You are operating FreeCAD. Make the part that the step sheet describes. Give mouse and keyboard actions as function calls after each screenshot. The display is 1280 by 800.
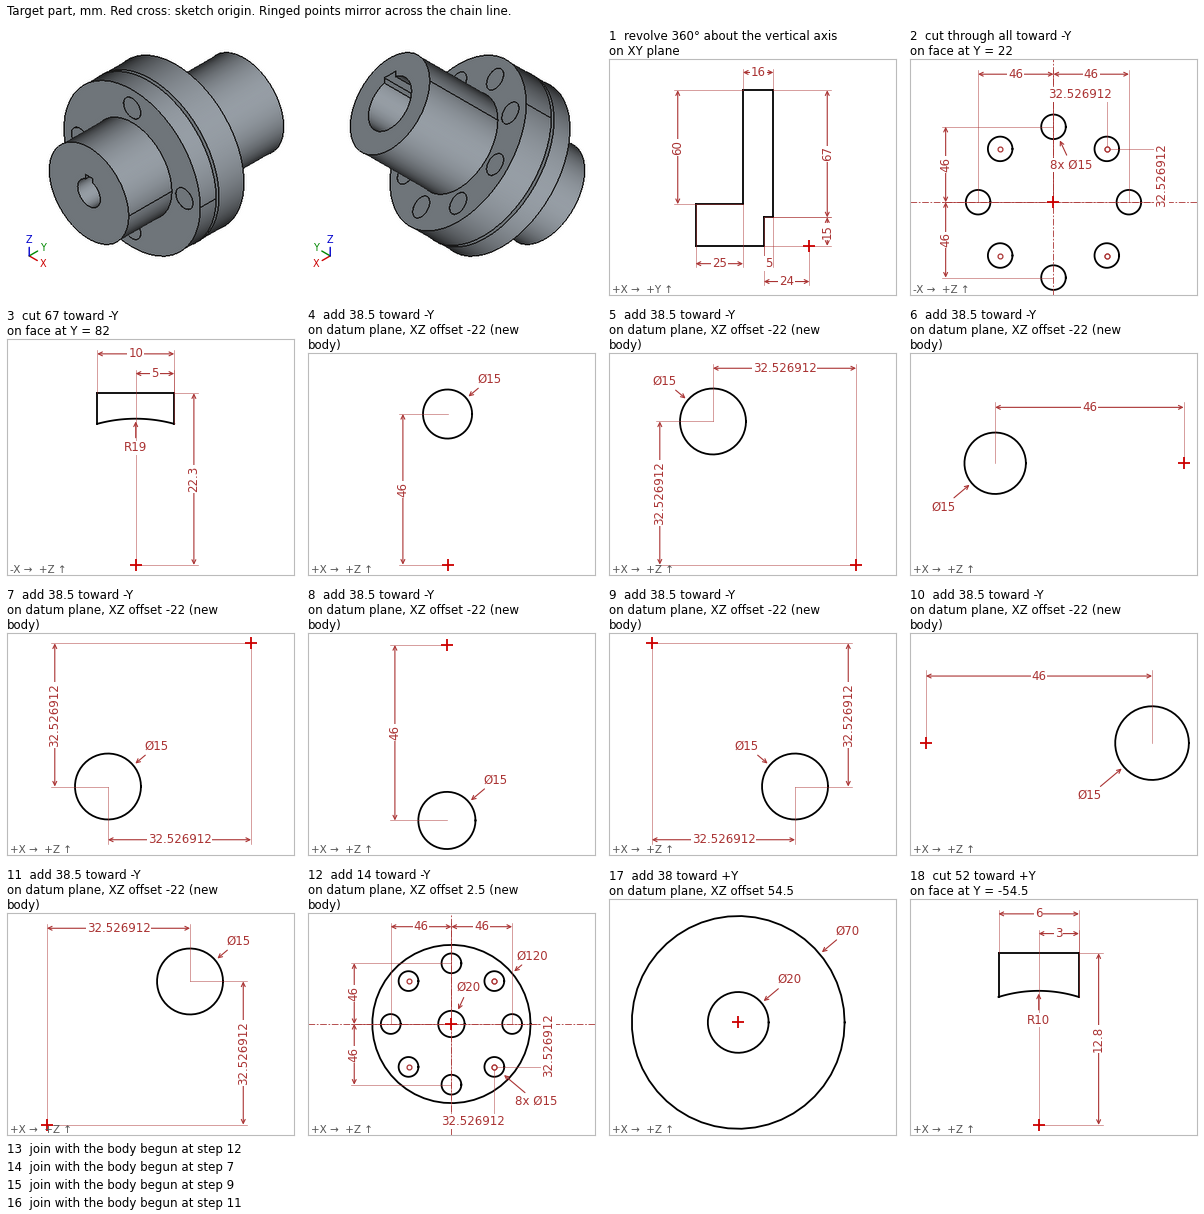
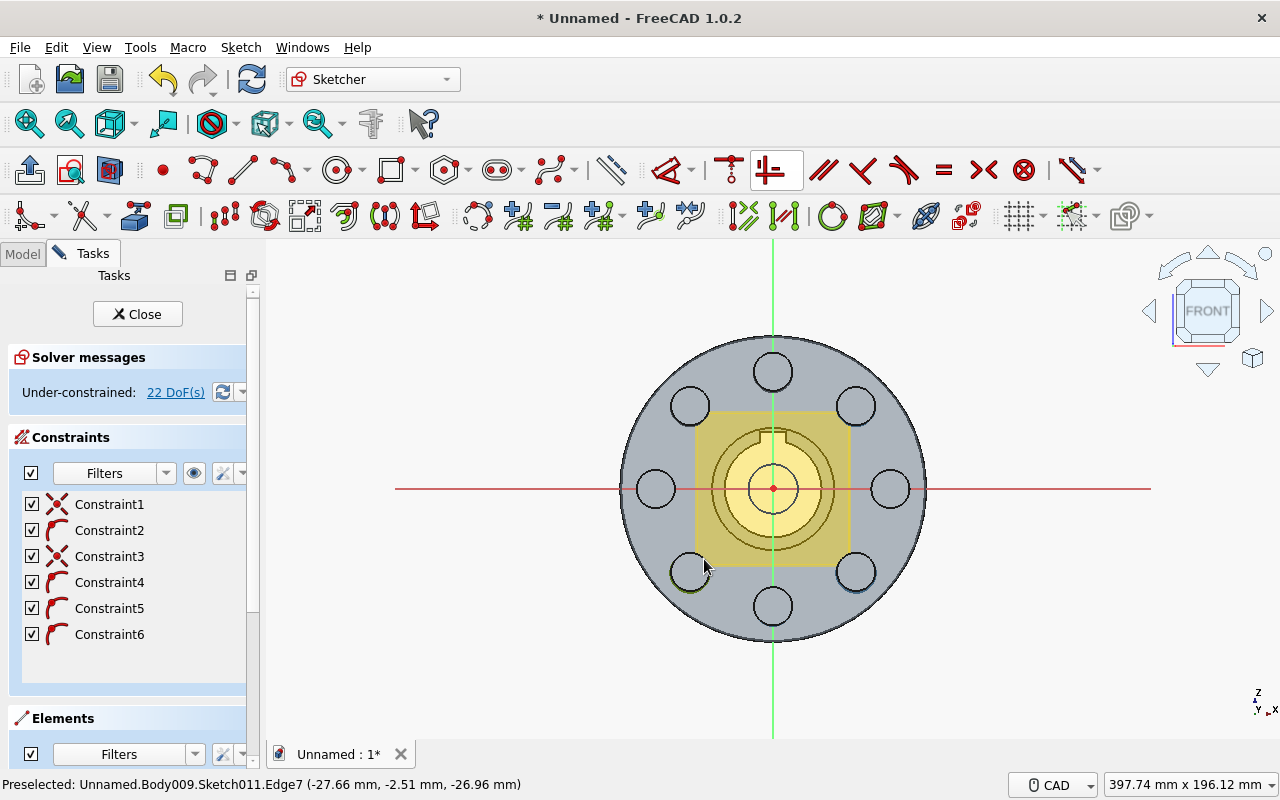
click(669, 476)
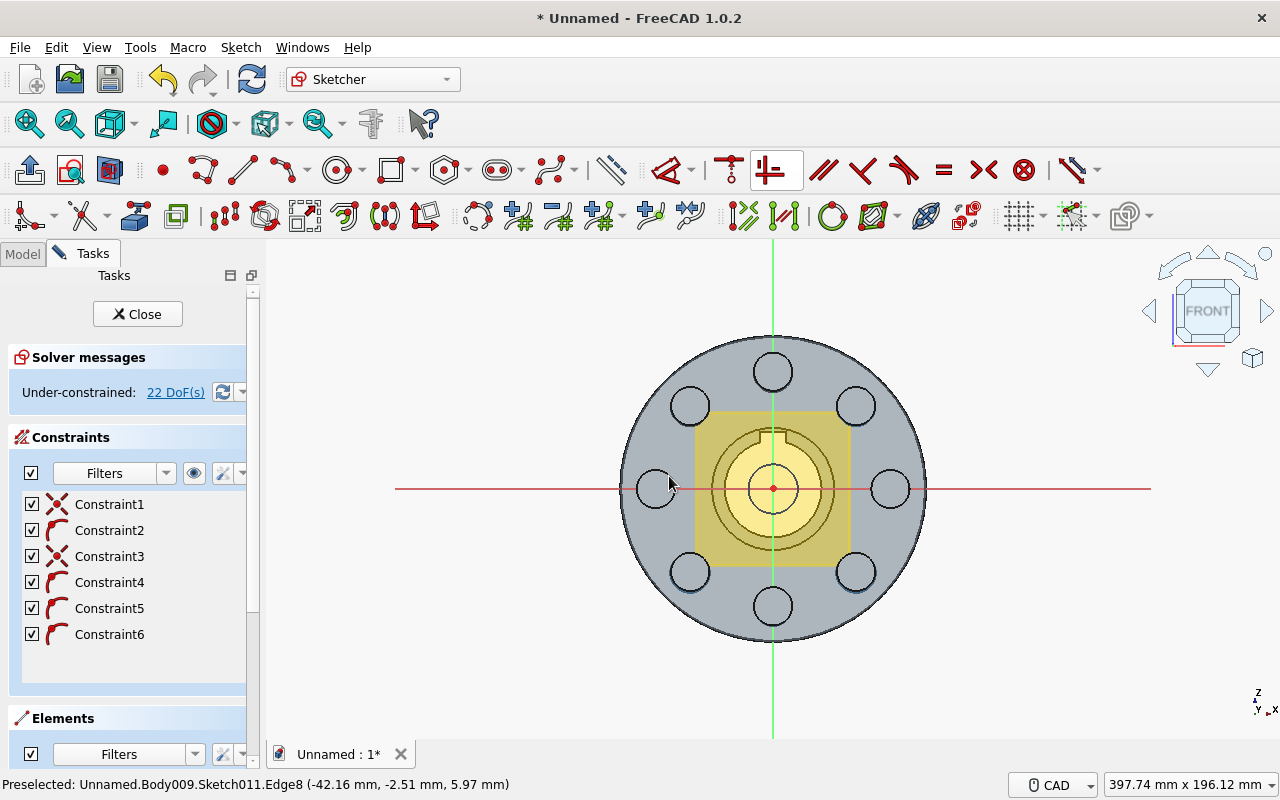
click(787, 359)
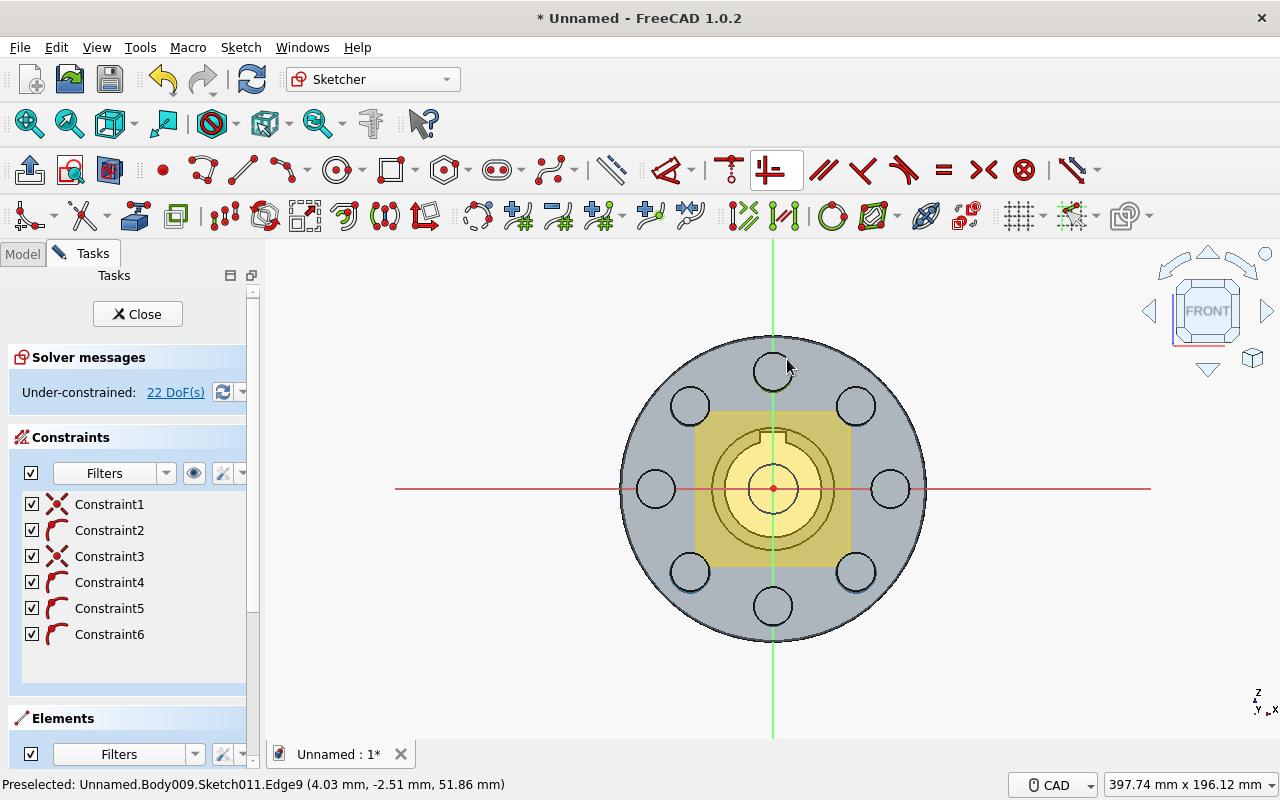
click(703, 393)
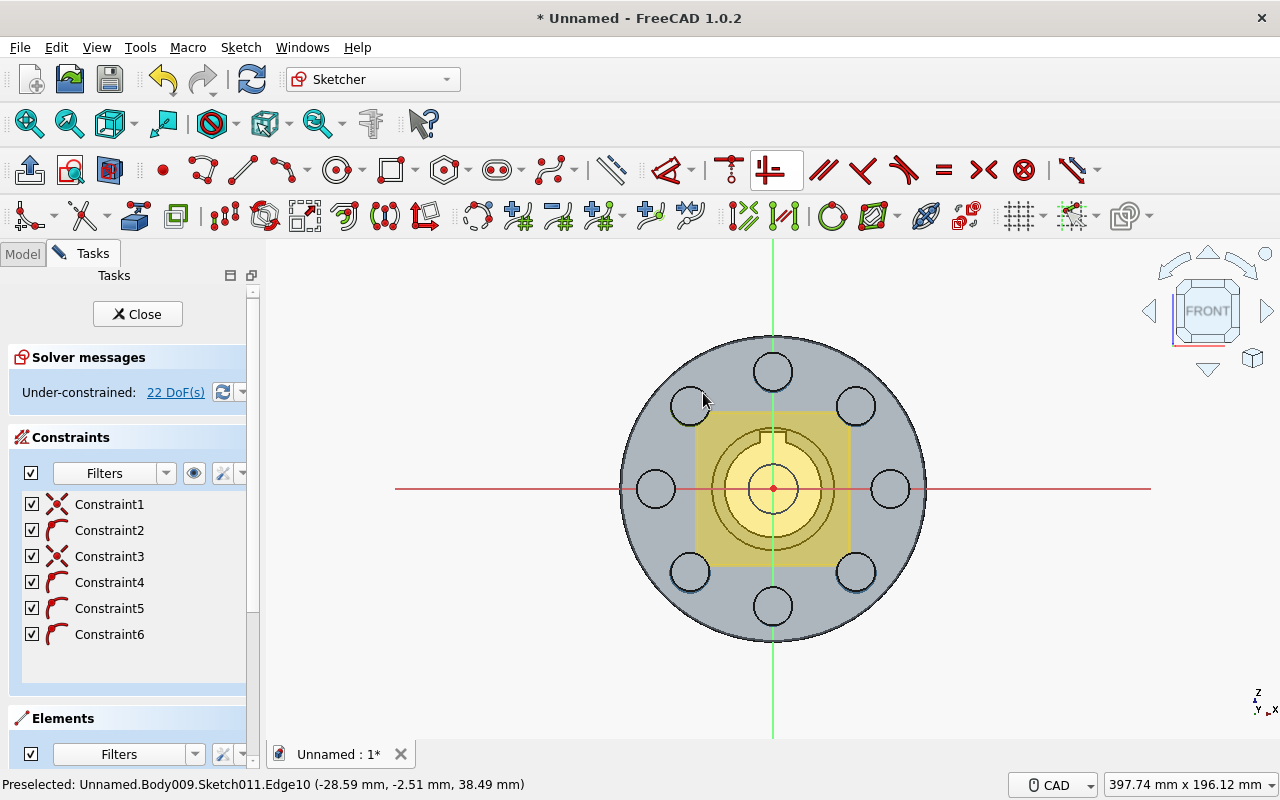
click(944, 170)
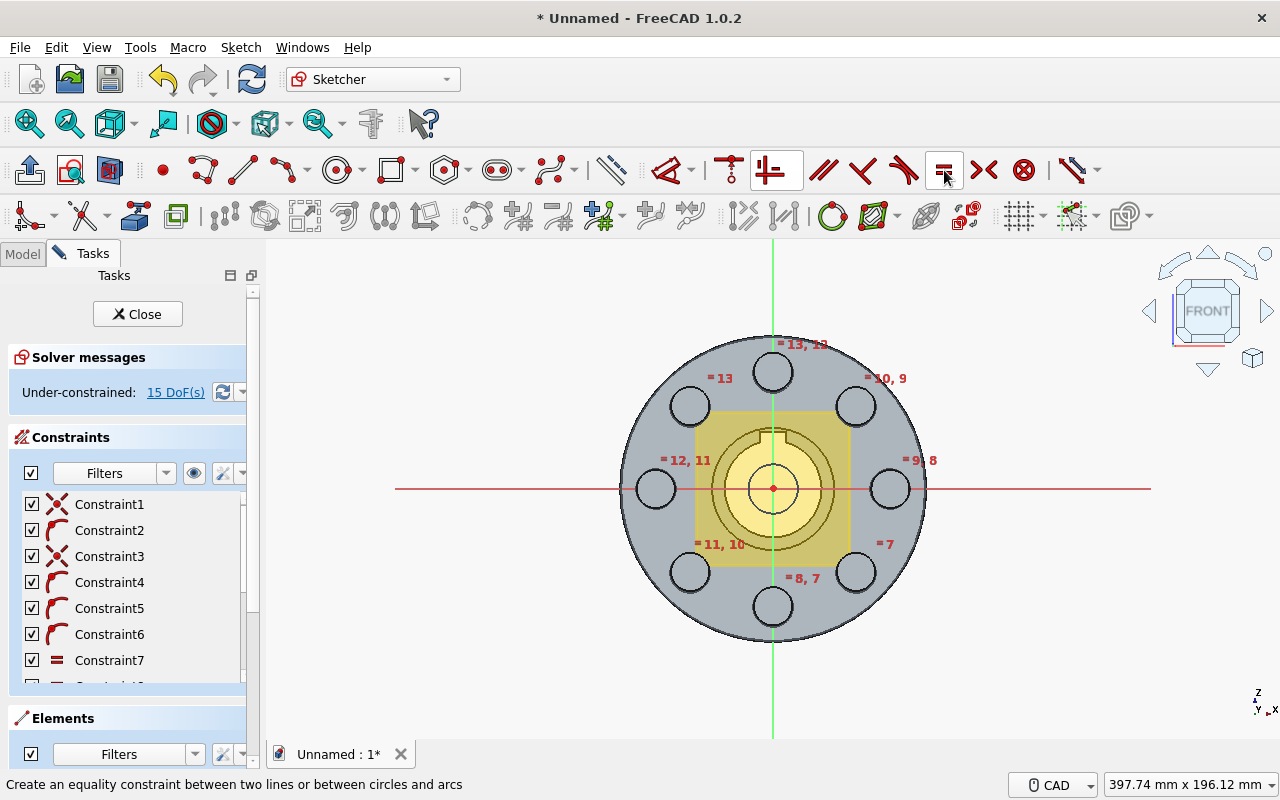
click(856, 573)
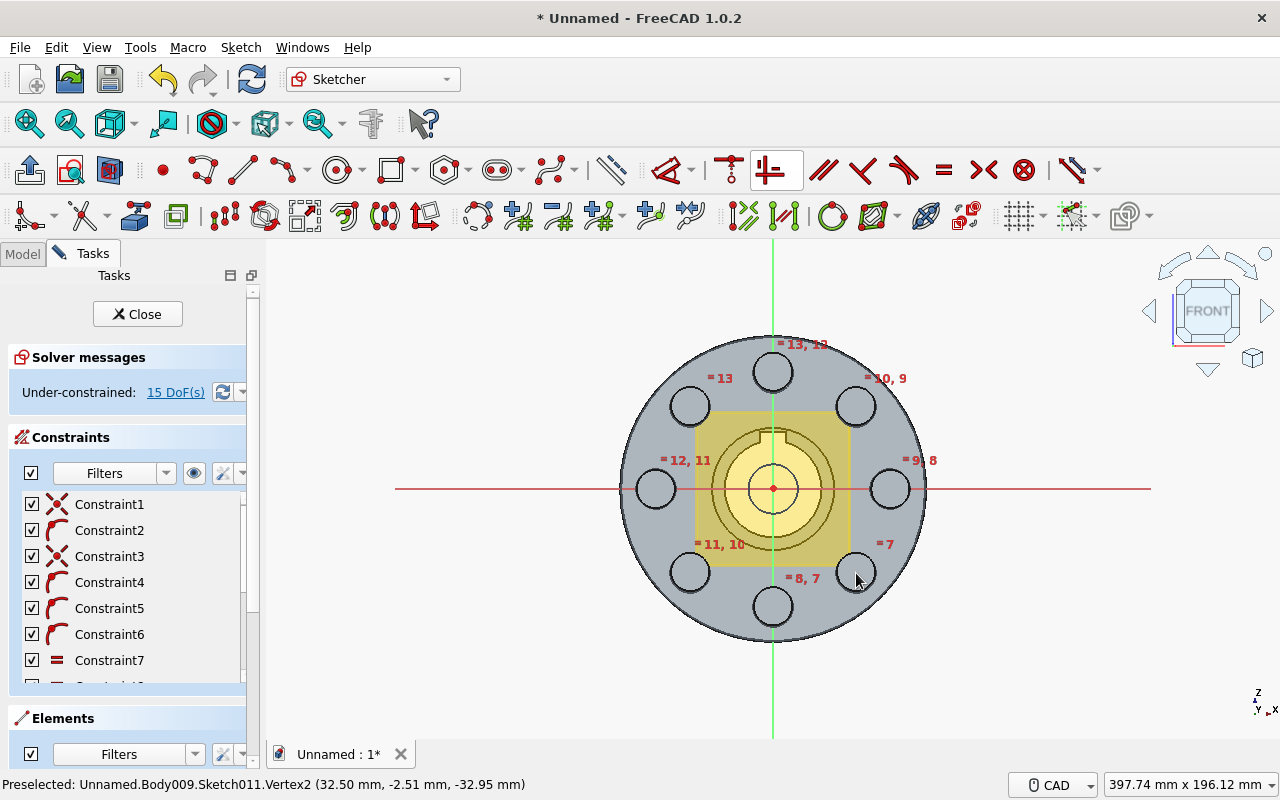
click(856, 407)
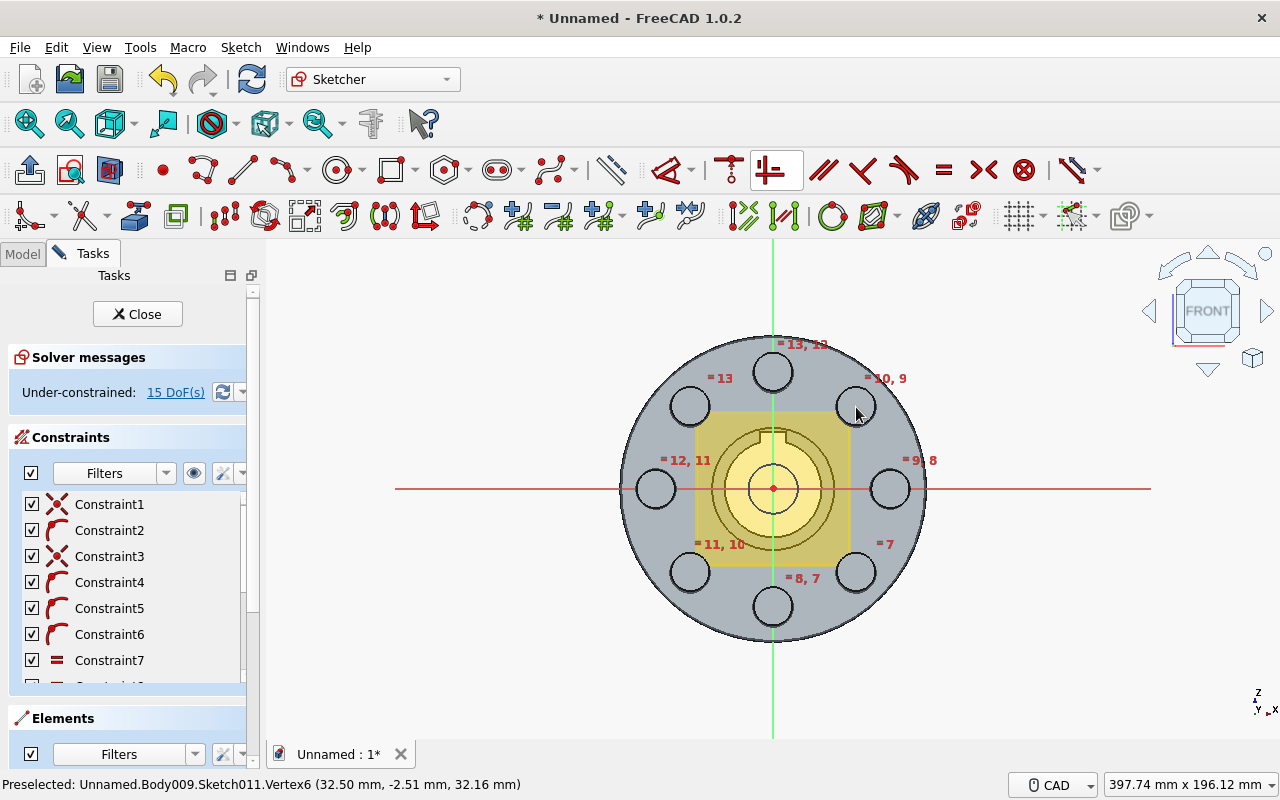
click(411, 489)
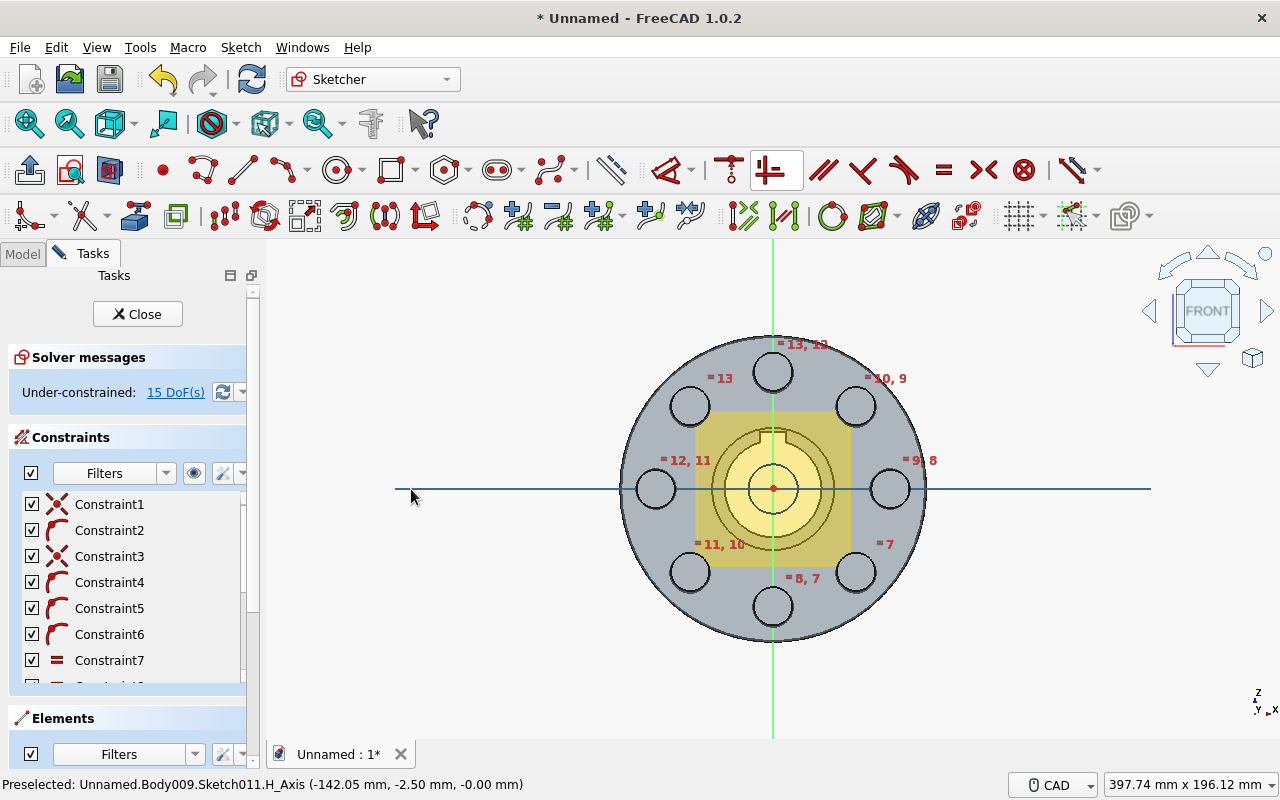
click(984, 170)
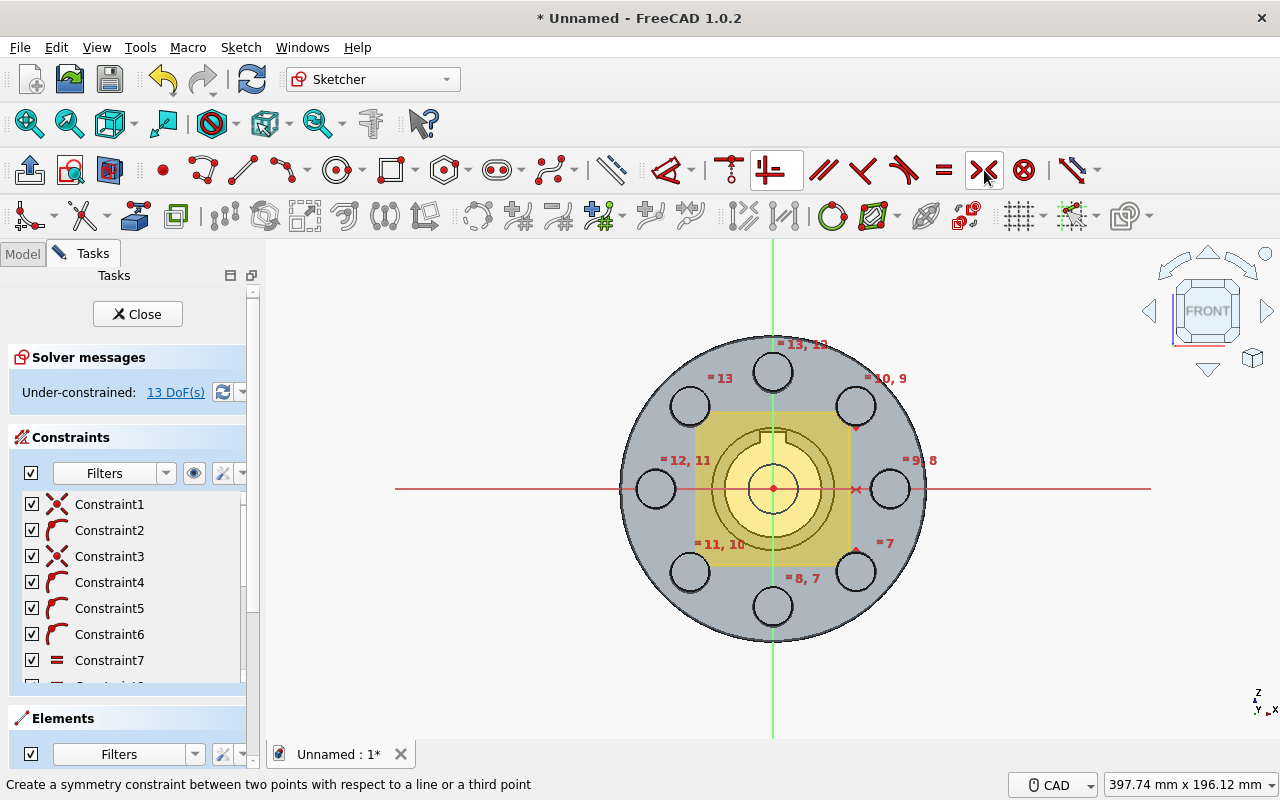
click(856, 572)